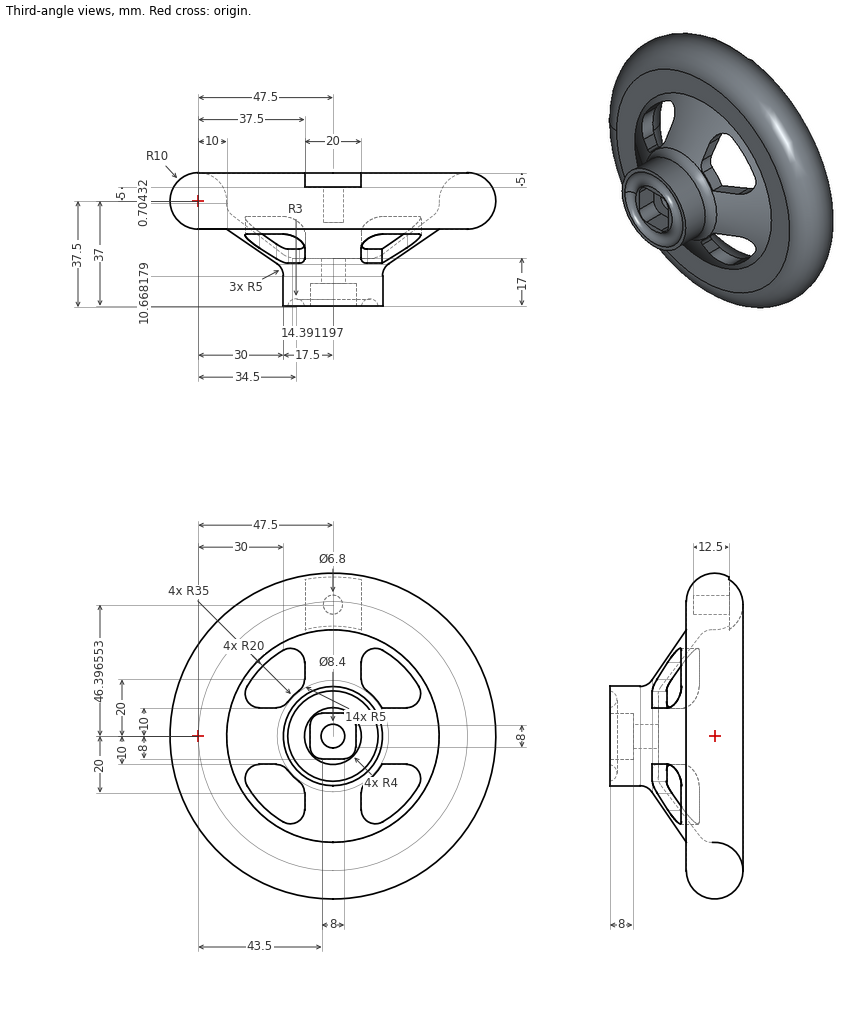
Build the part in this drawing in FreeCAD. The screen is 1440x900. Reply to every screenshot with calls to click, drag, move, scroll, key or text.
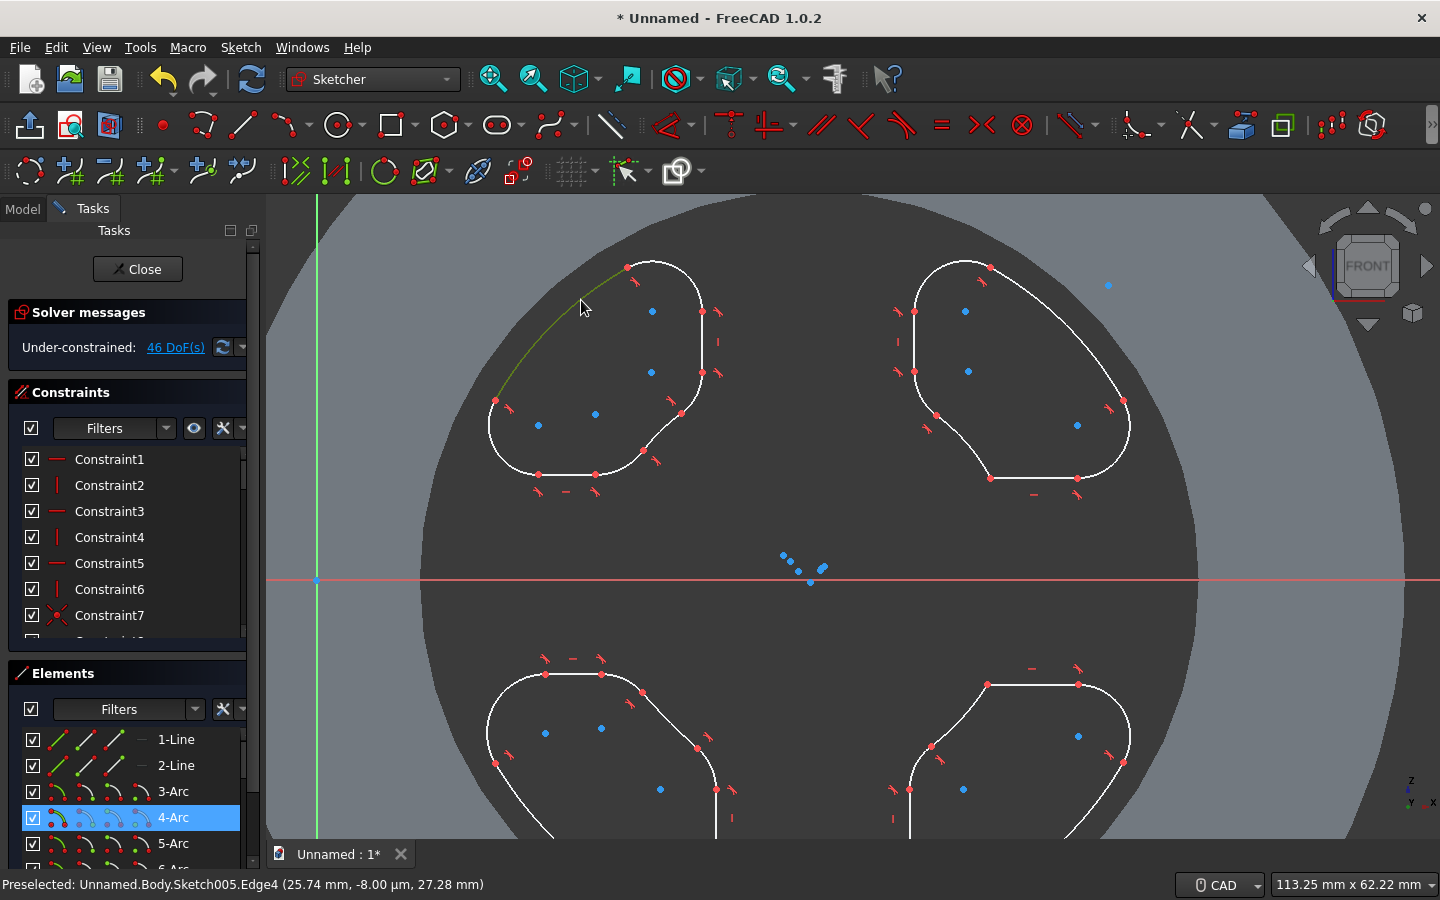
click(669, 424)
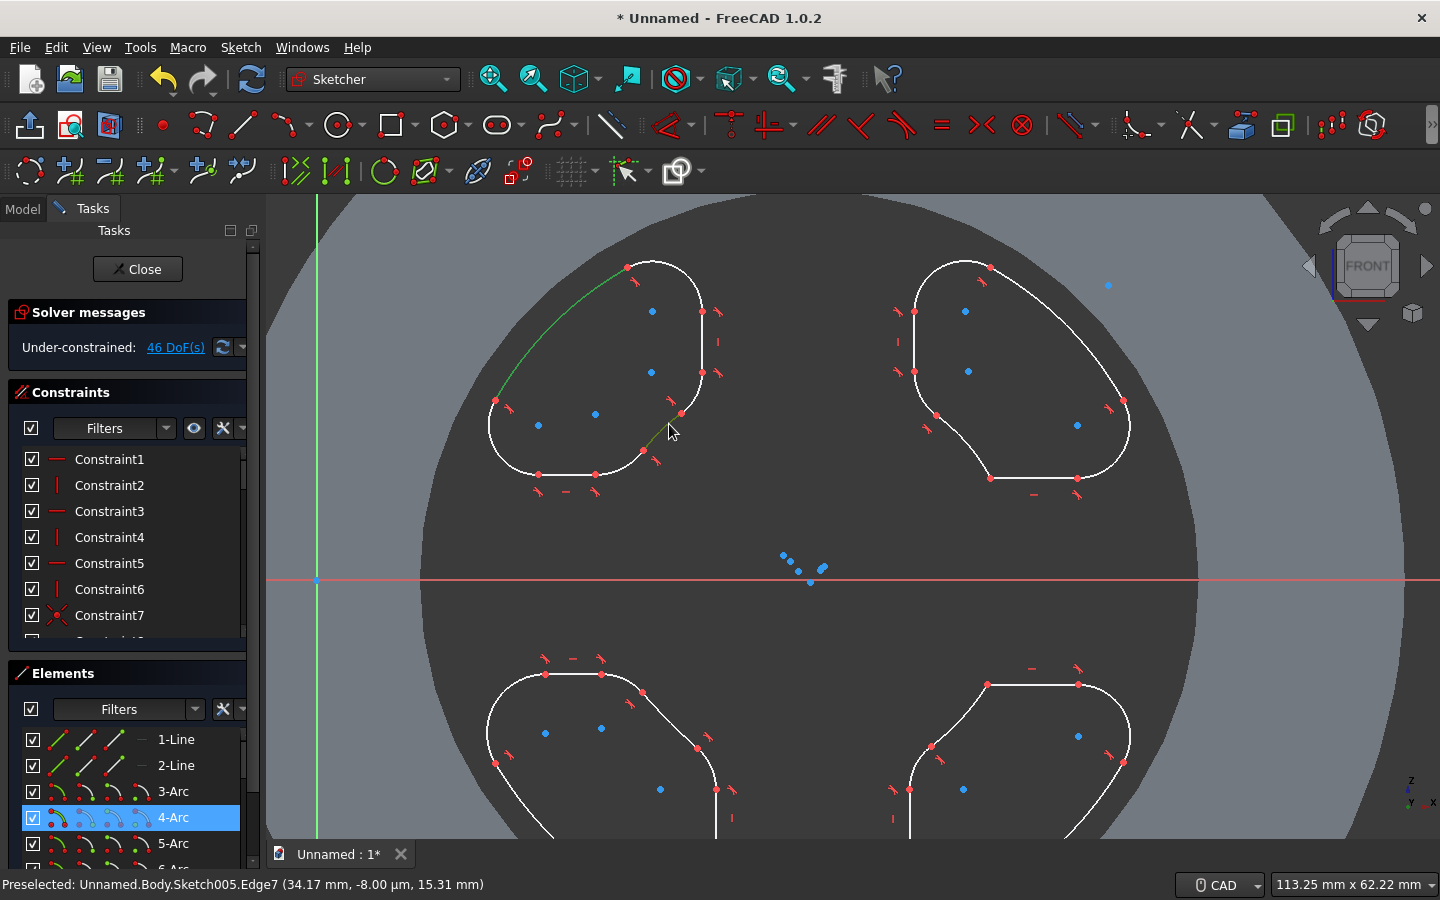
click(730, 126)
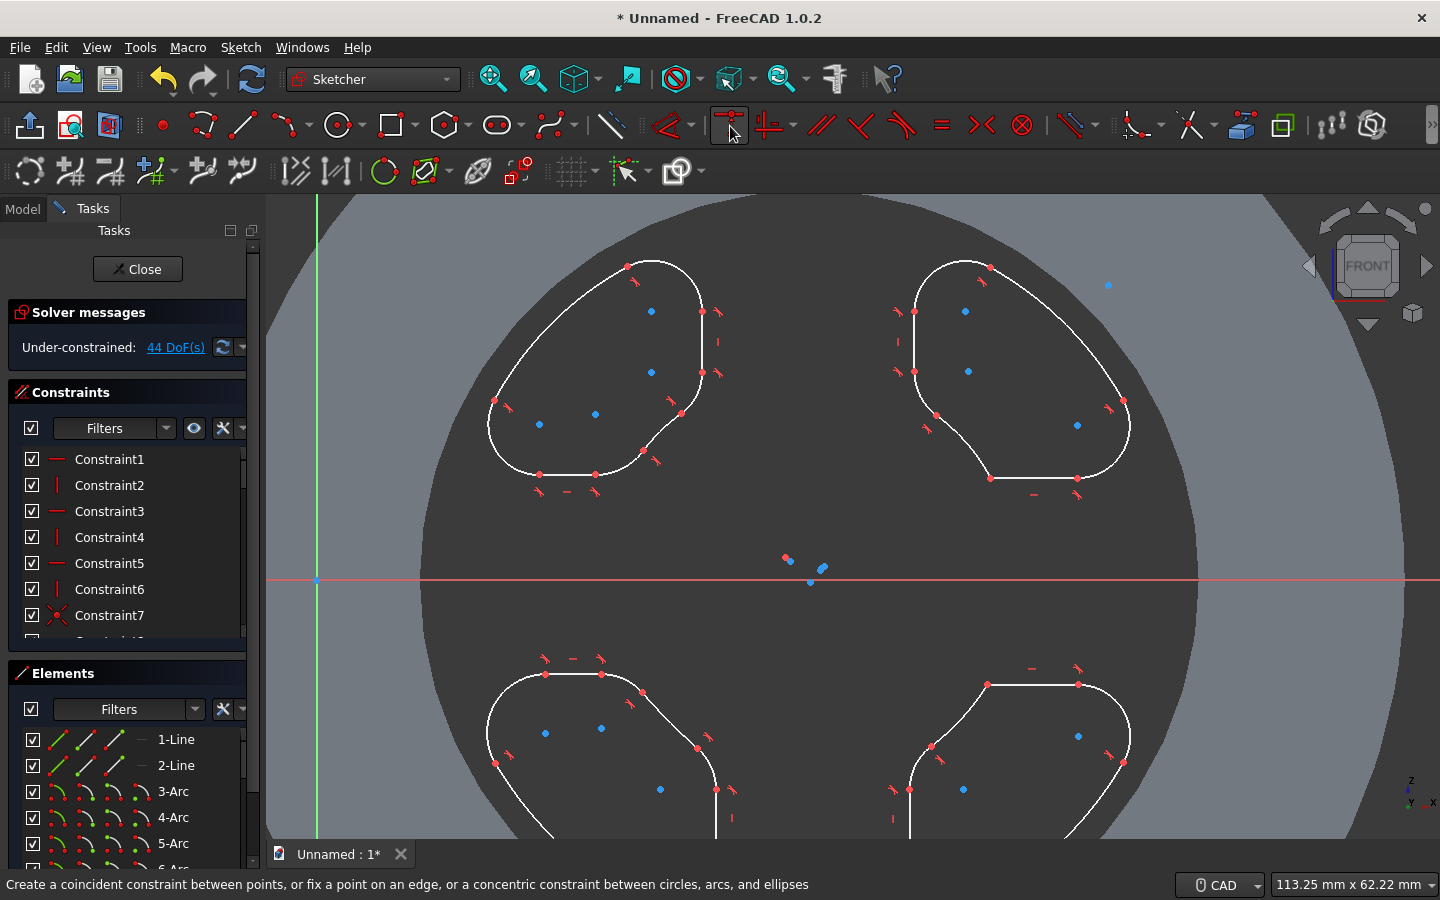
click(580, 298)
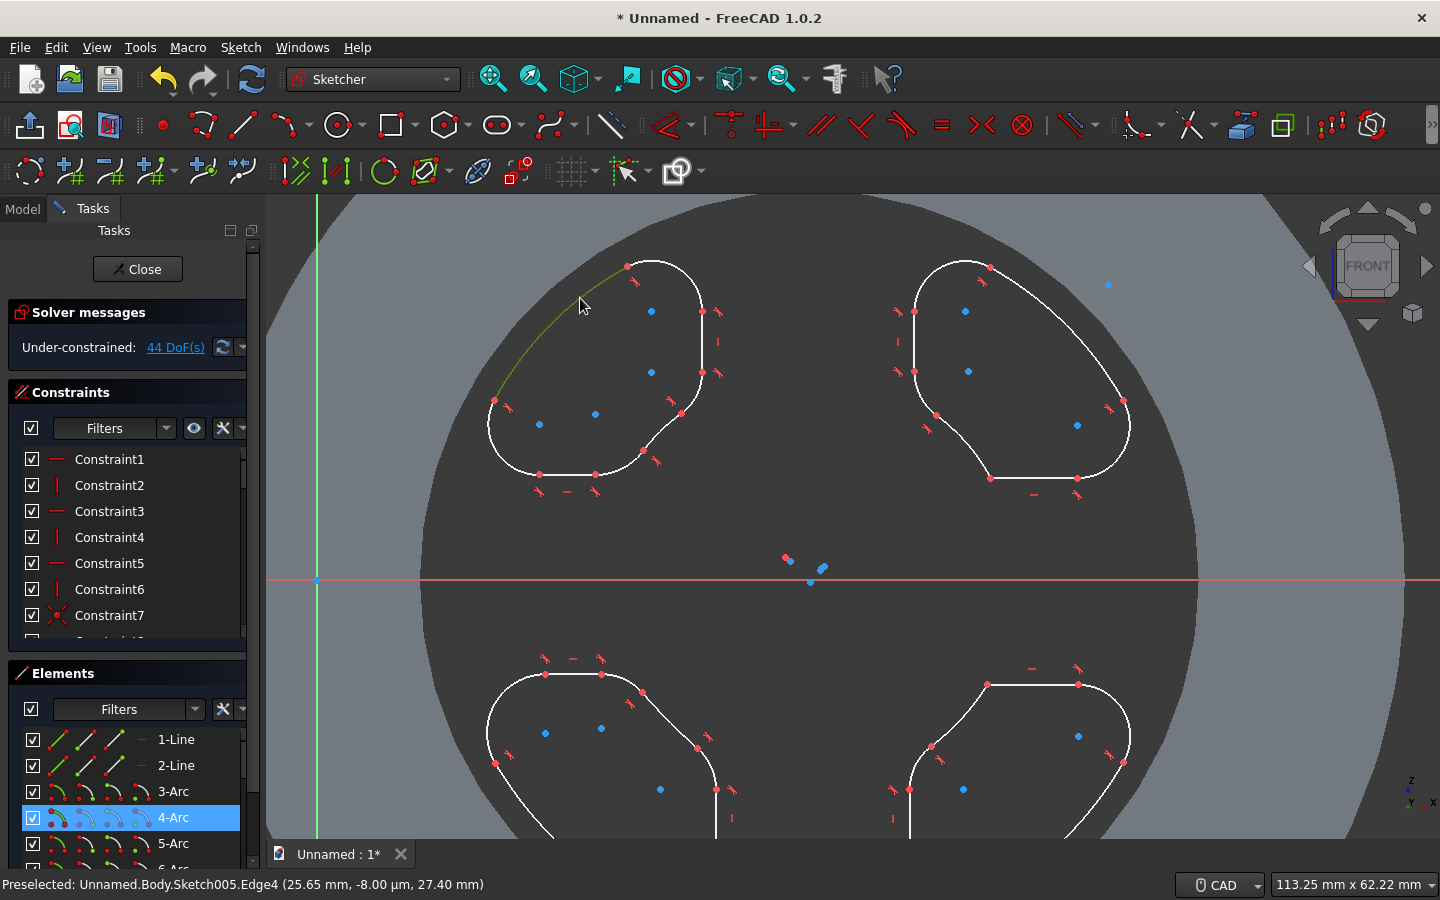
click(658, 710)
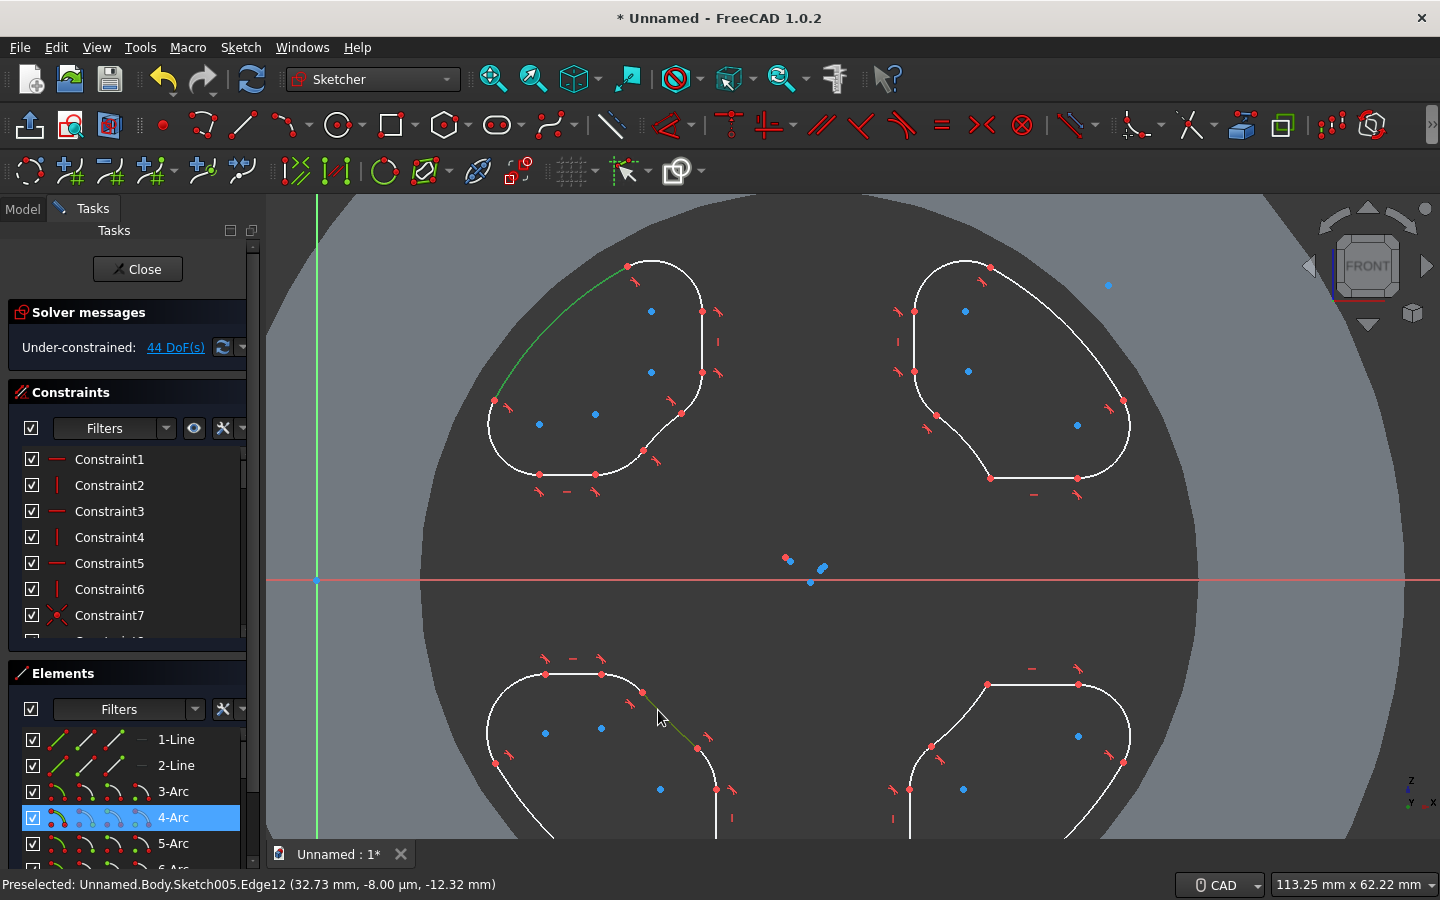
click(730, 126)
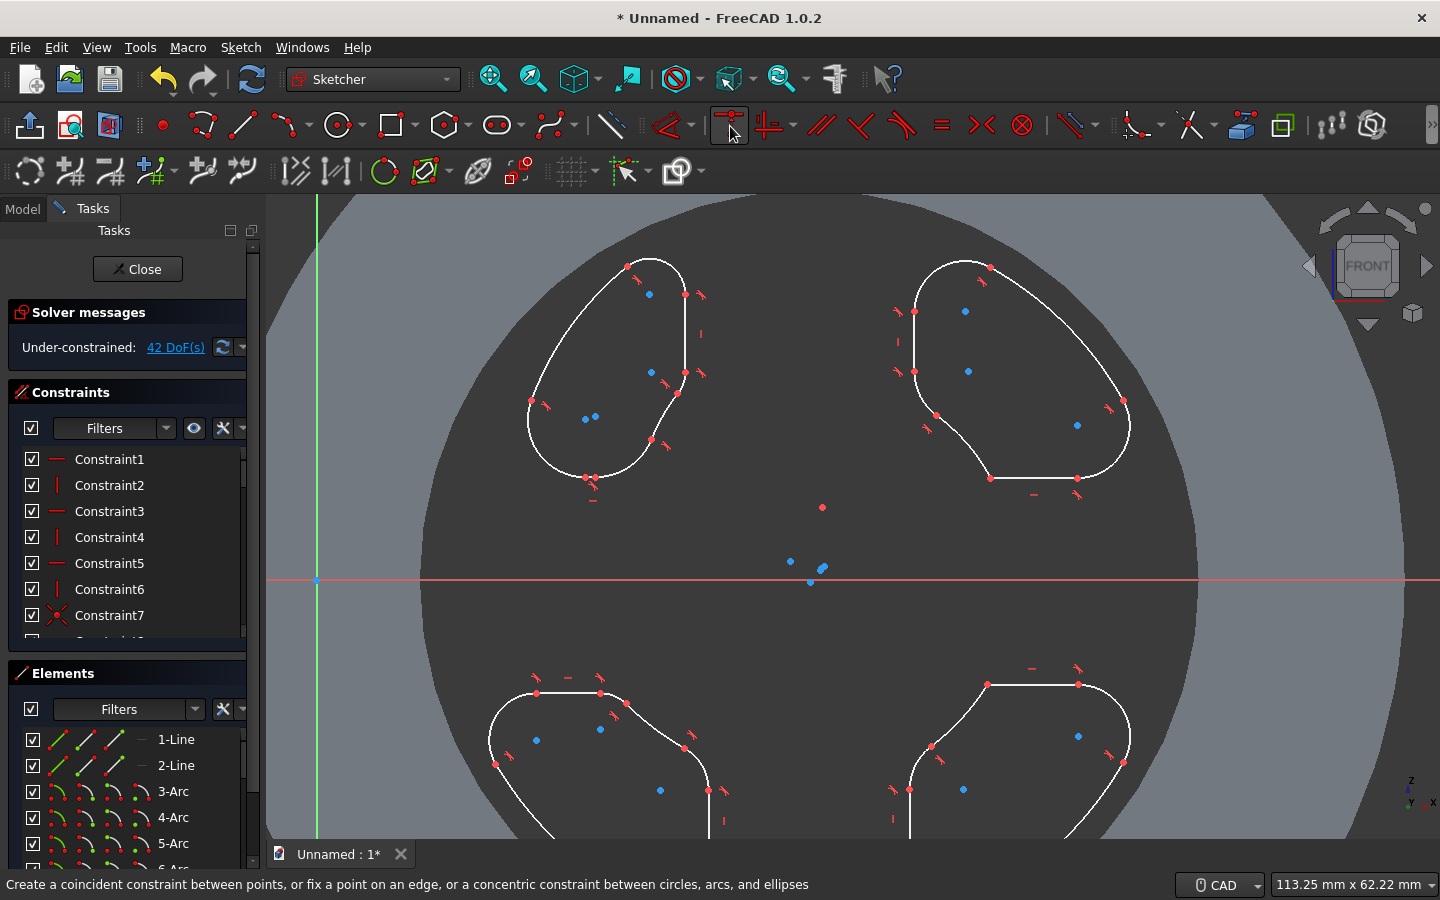
click(591, 301)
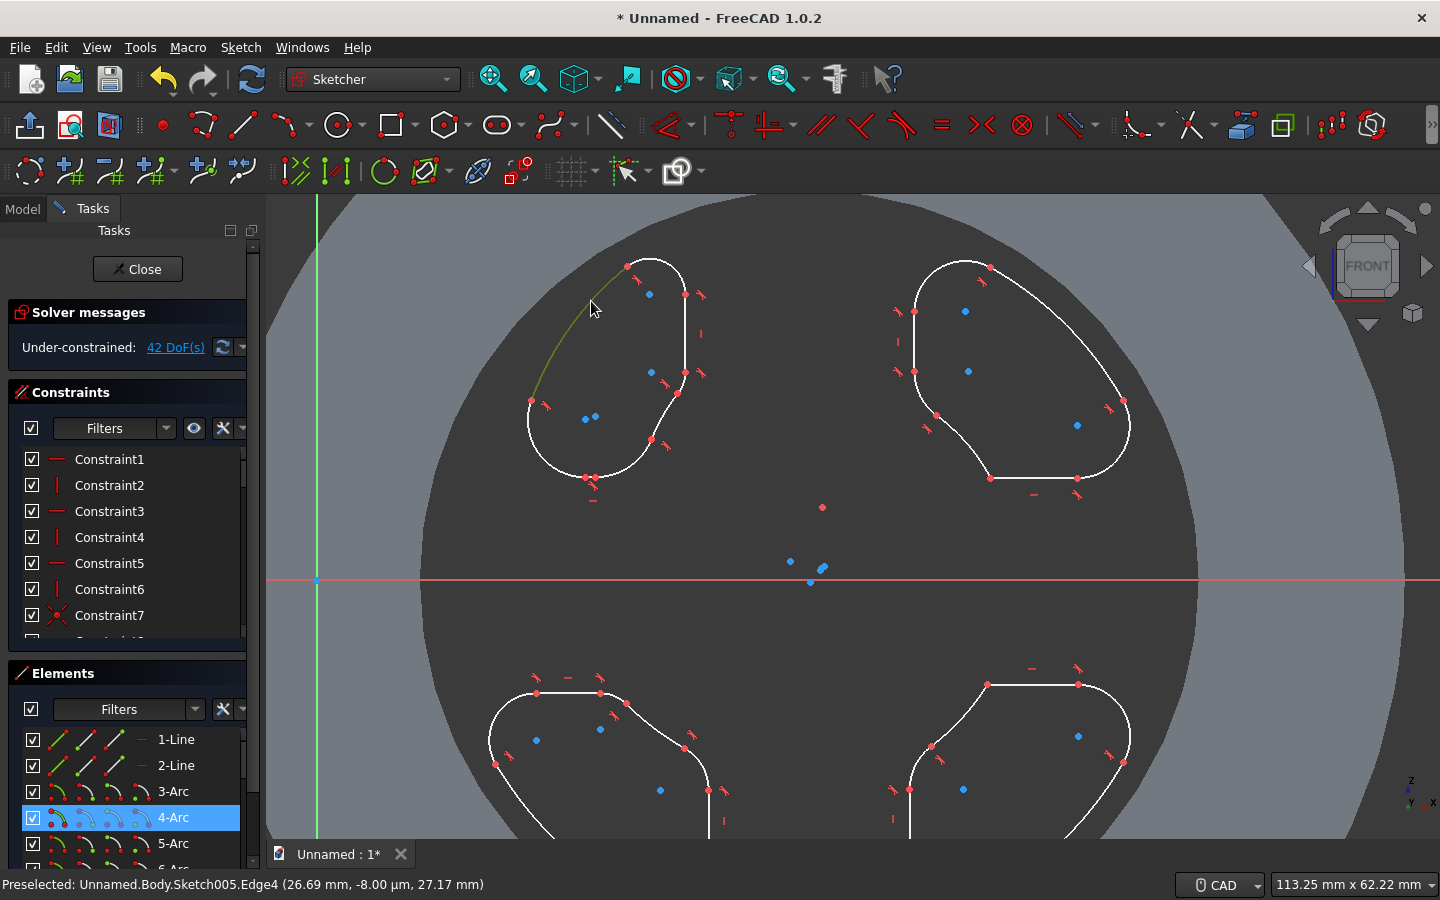
click(529, 811)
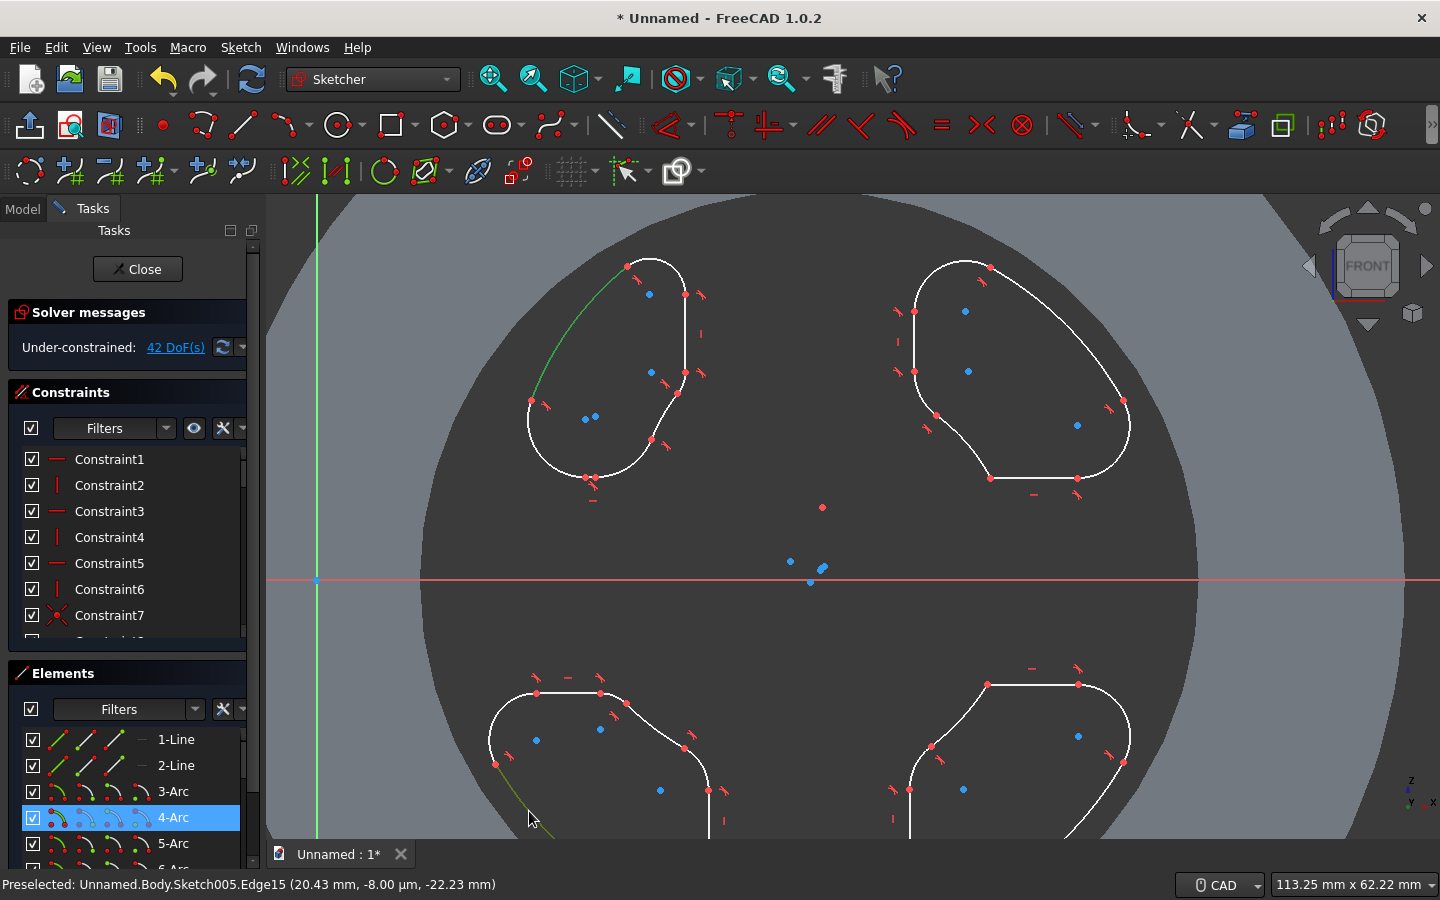
click(730, 126)